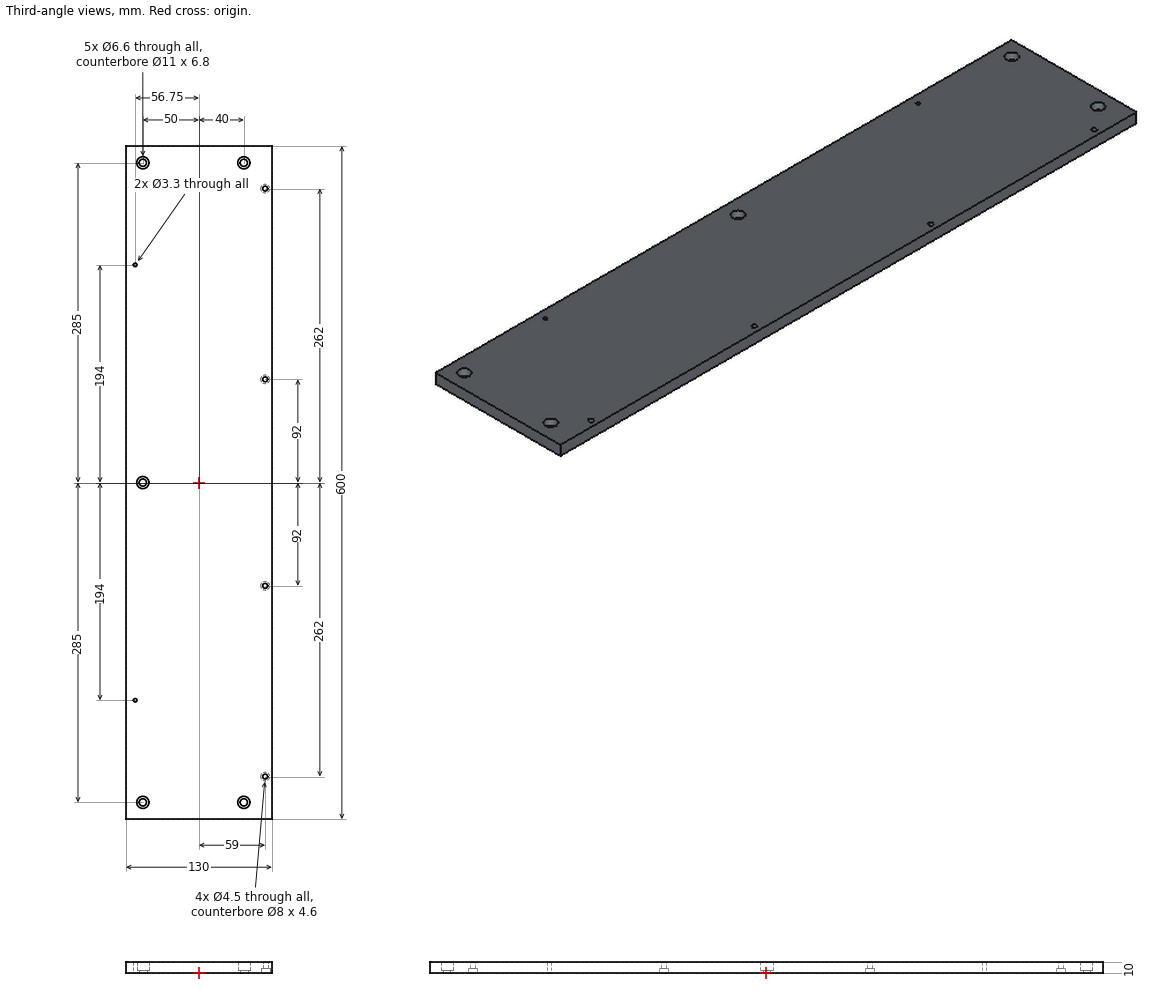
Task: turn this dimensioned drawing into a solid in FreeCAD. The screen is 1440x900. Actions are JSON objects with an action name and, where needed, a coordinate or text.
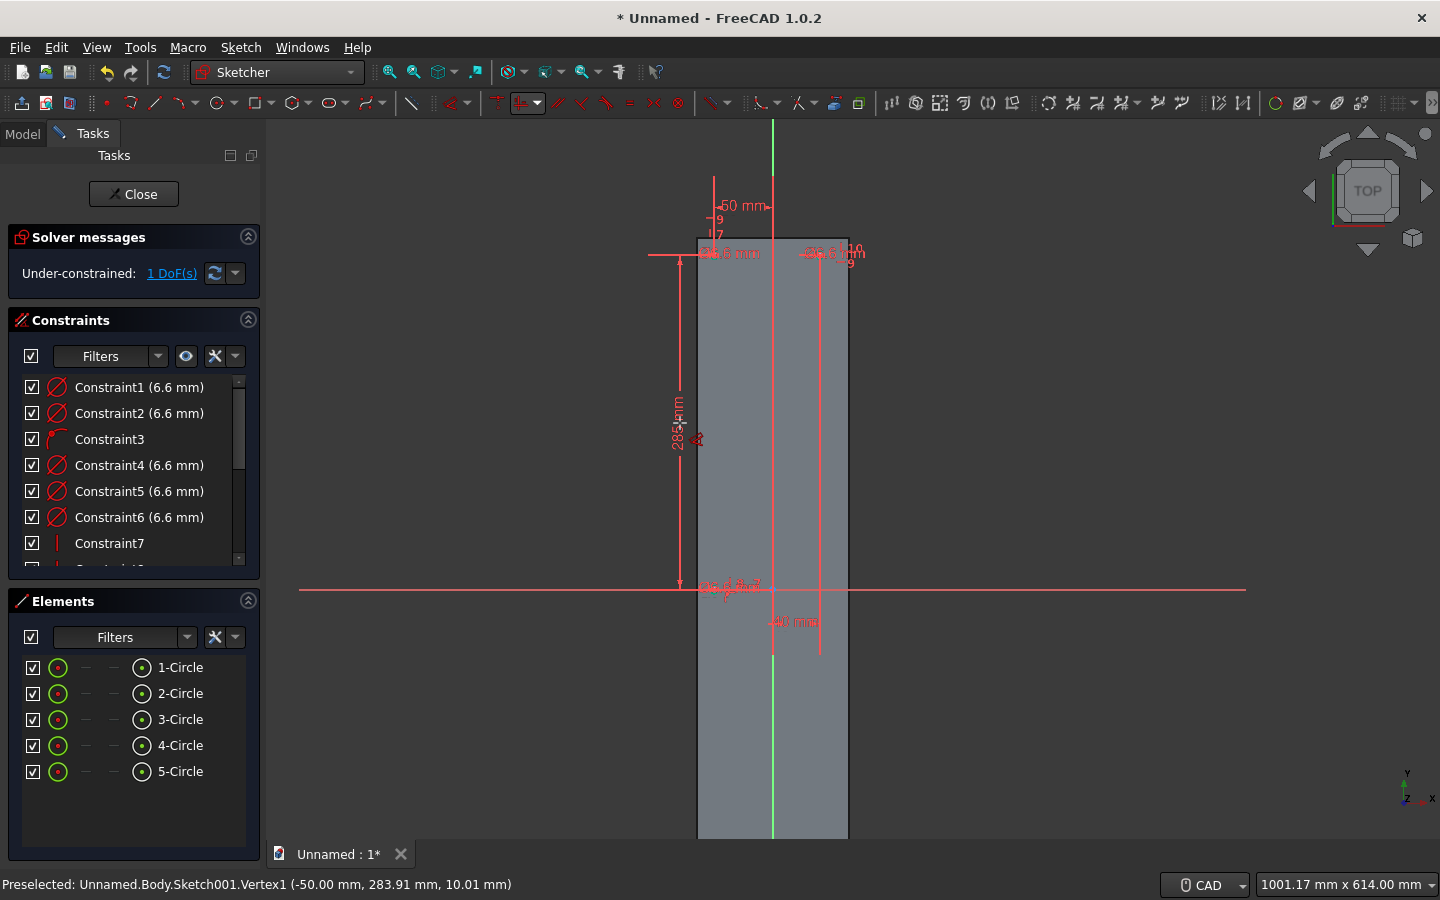
{"action": "scroll", "coordinate": [820, 254], "scroll_direction": "down", "scroll_amount": 2}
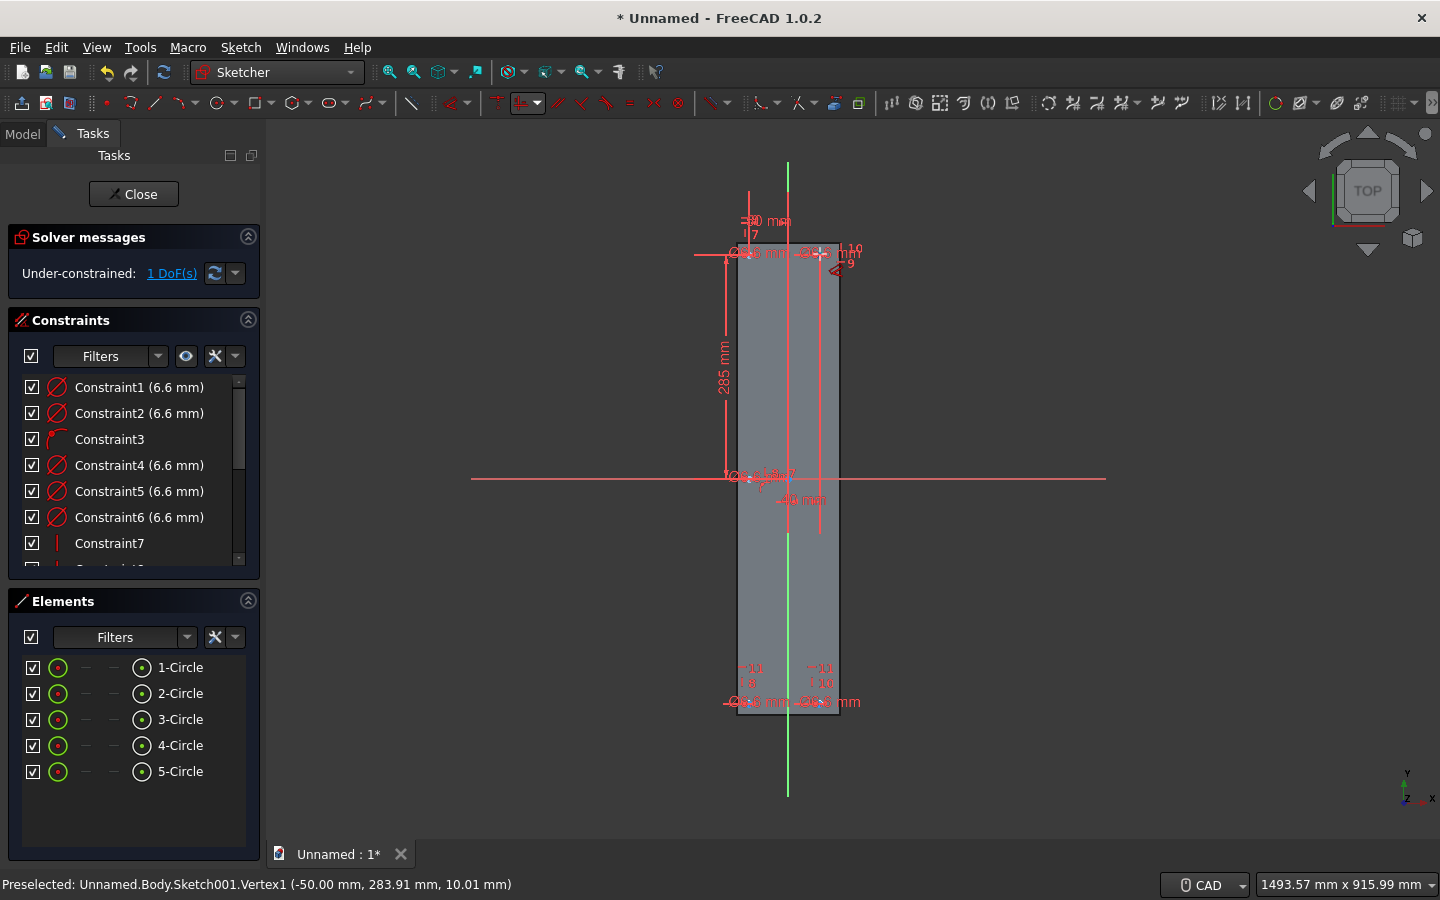
{"action": "left_click", "coordinate": [749, 704]}
{"action": "left_click", "coordinate": [715, 592]}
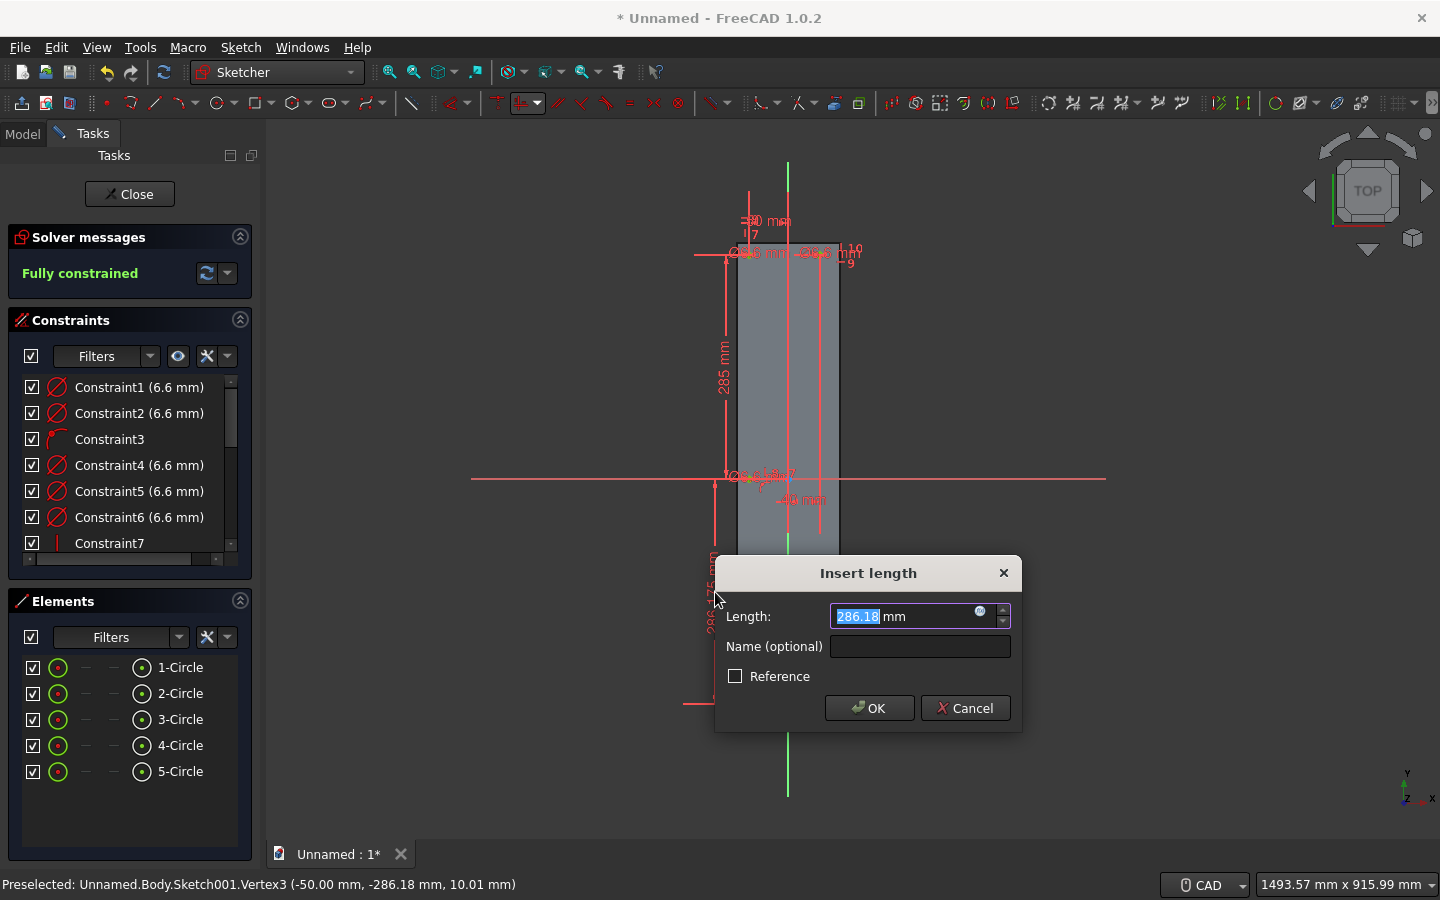
{"action": "type", "text": "285"}
{"action": "key", "text": "Return"}
{"action": "key", "text": "Escape"}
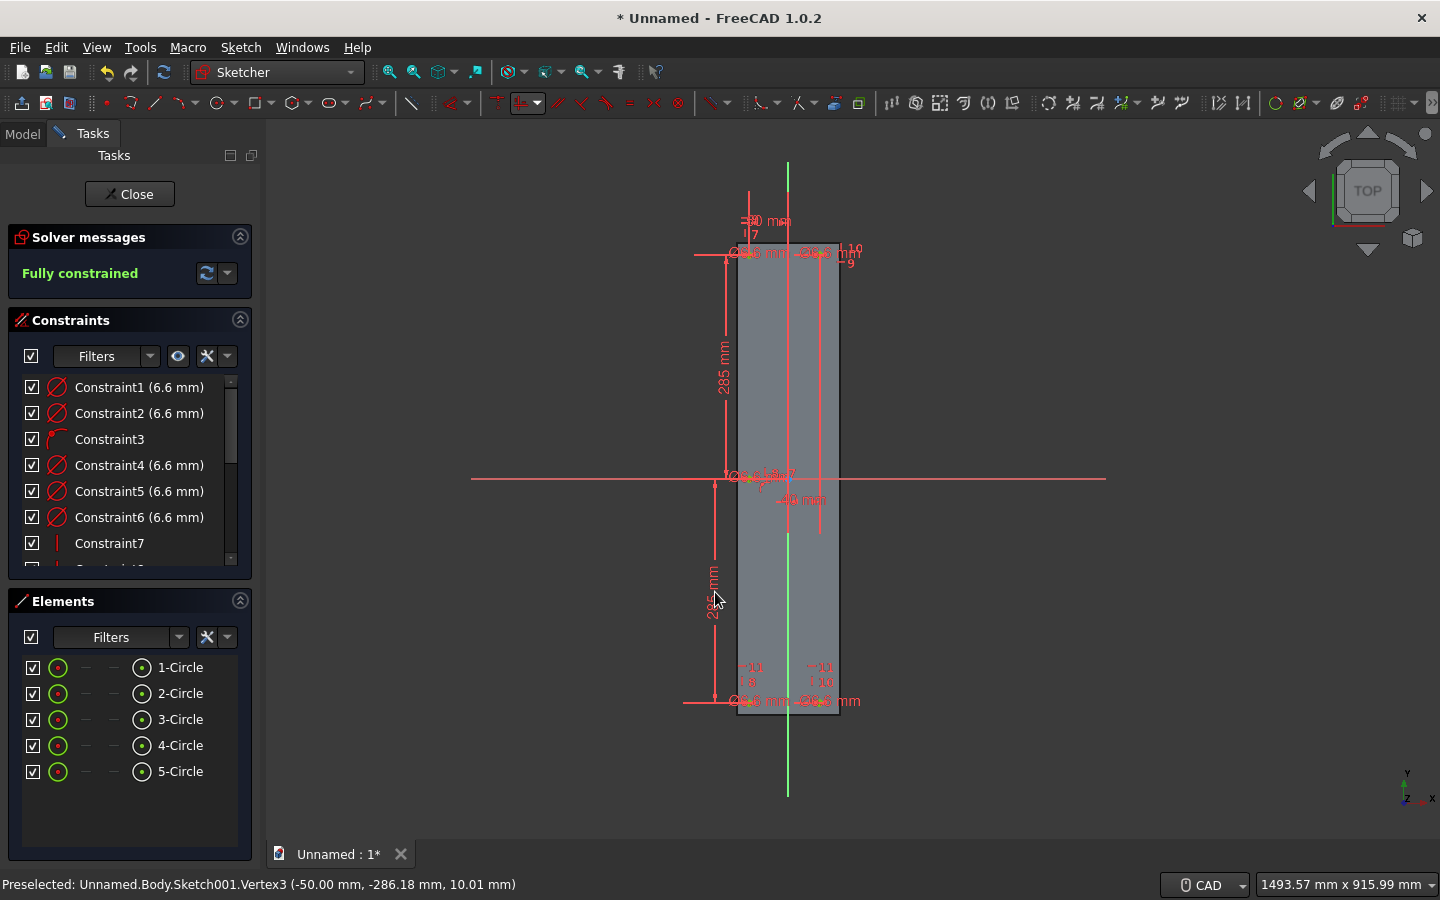
{"action": "left_click", "coordinate": [130, 194]}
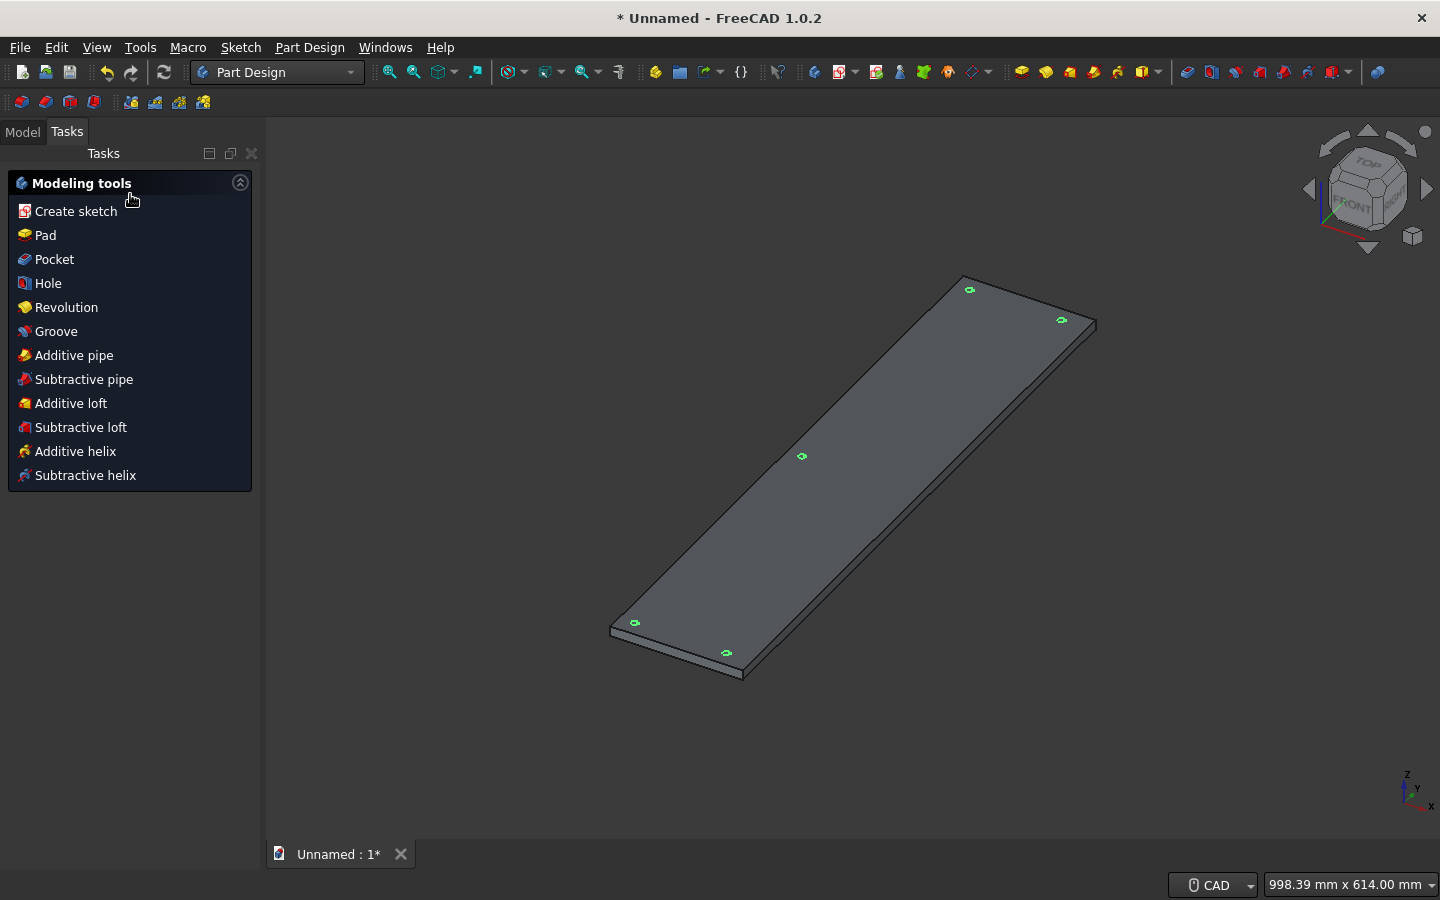
{"action": "left_click", "coordinate": [1212, 72]}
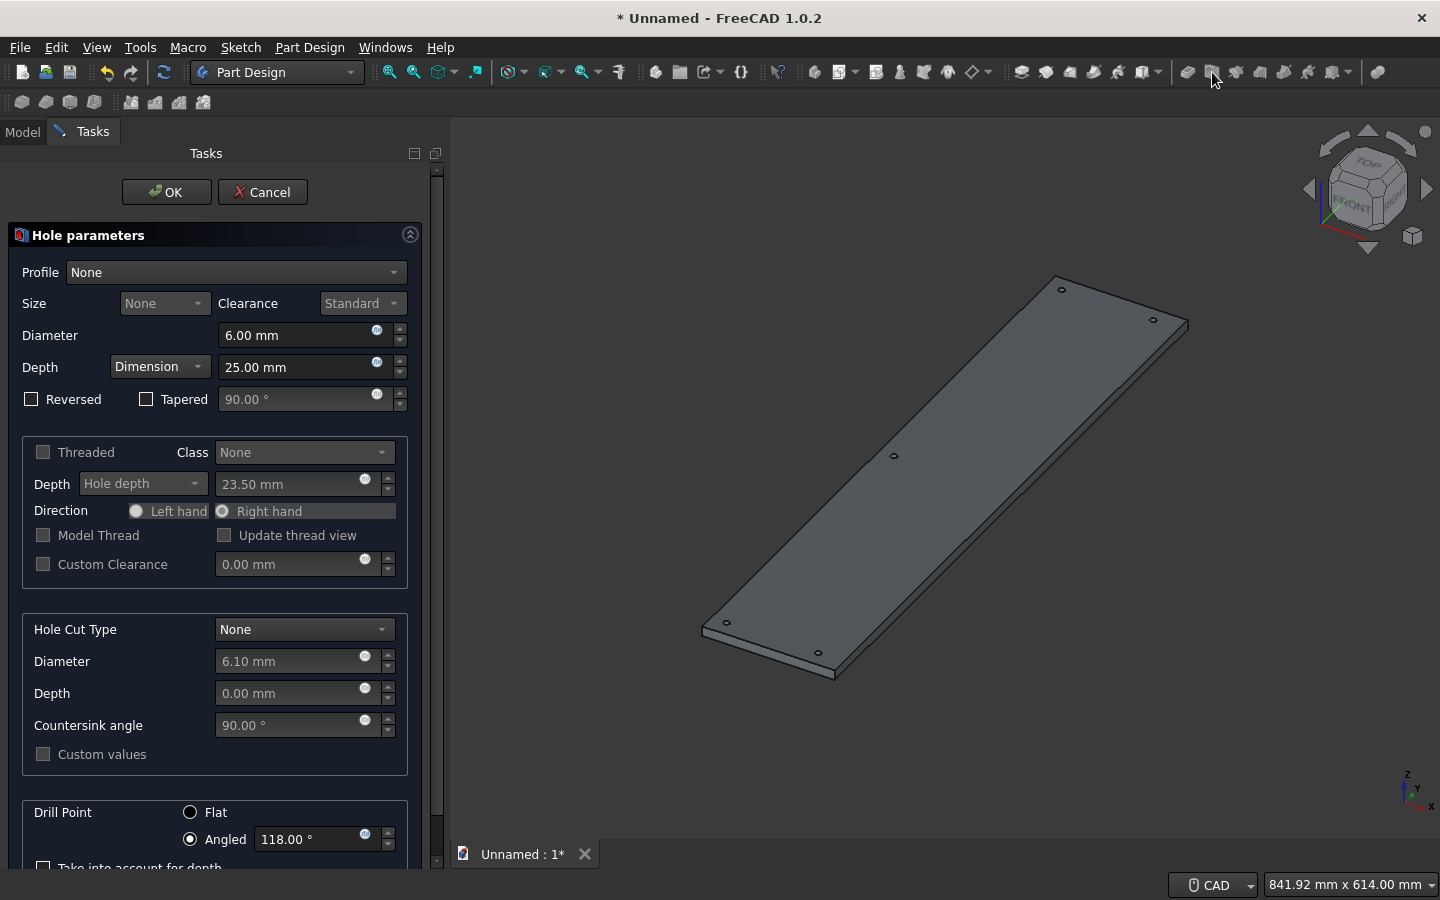
{"action": "triple_click", "coordinate": [305, 335]}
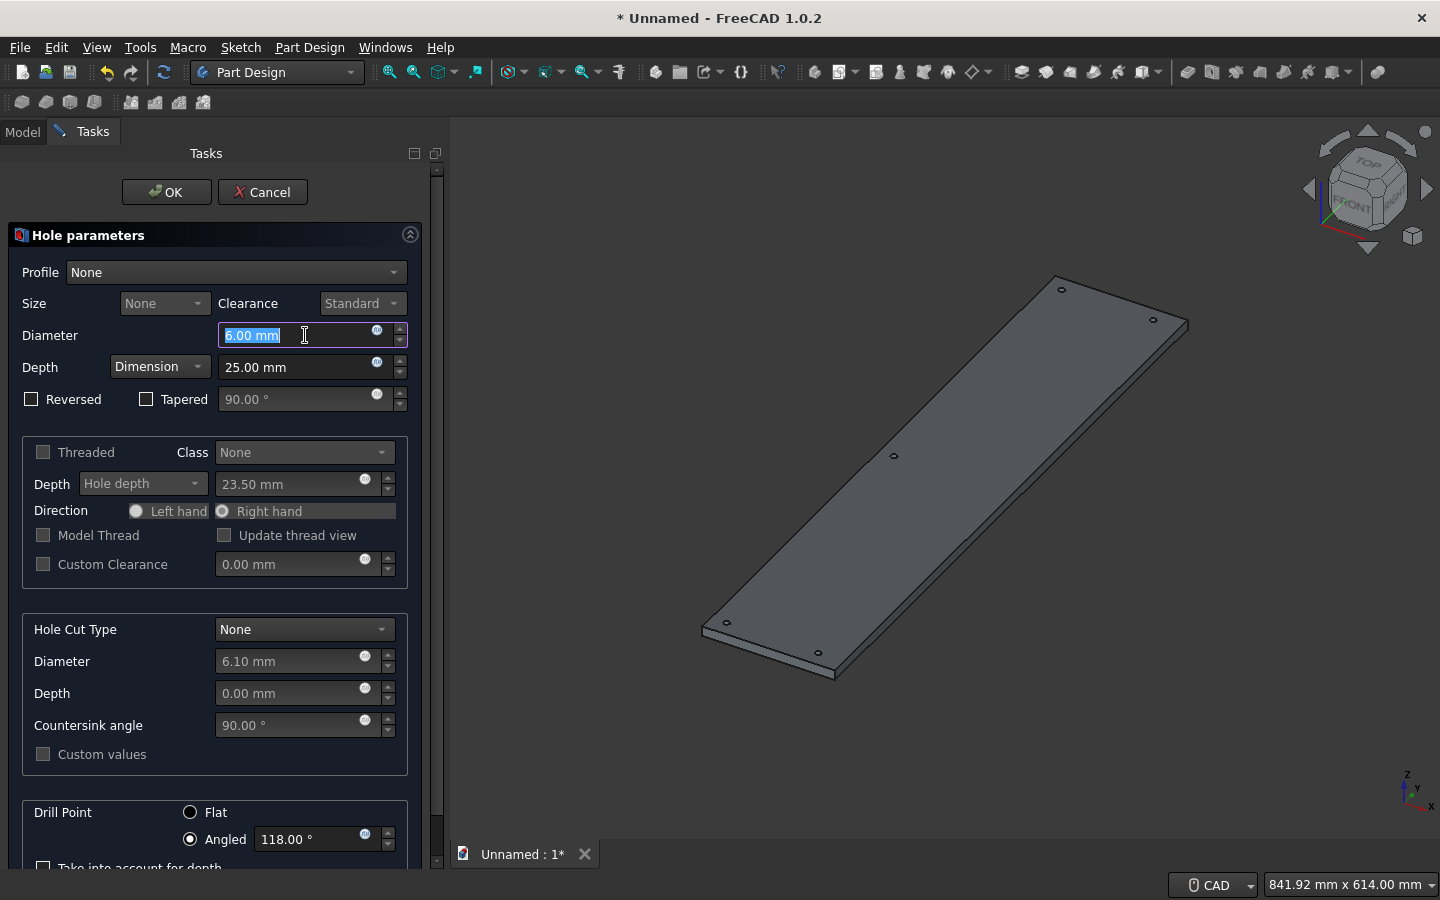
{"action": "type", "text": "6.6"}
{"action": "key", "text": "Tab"}